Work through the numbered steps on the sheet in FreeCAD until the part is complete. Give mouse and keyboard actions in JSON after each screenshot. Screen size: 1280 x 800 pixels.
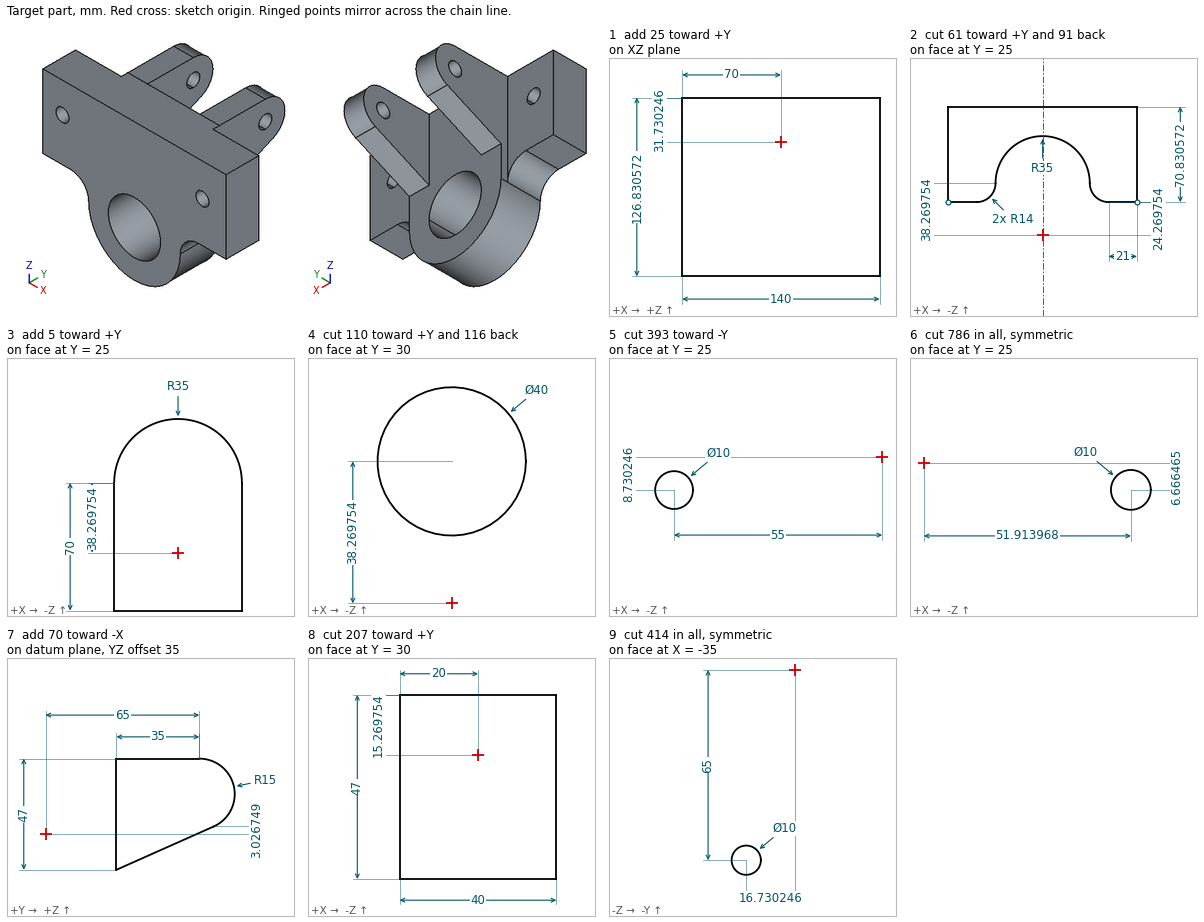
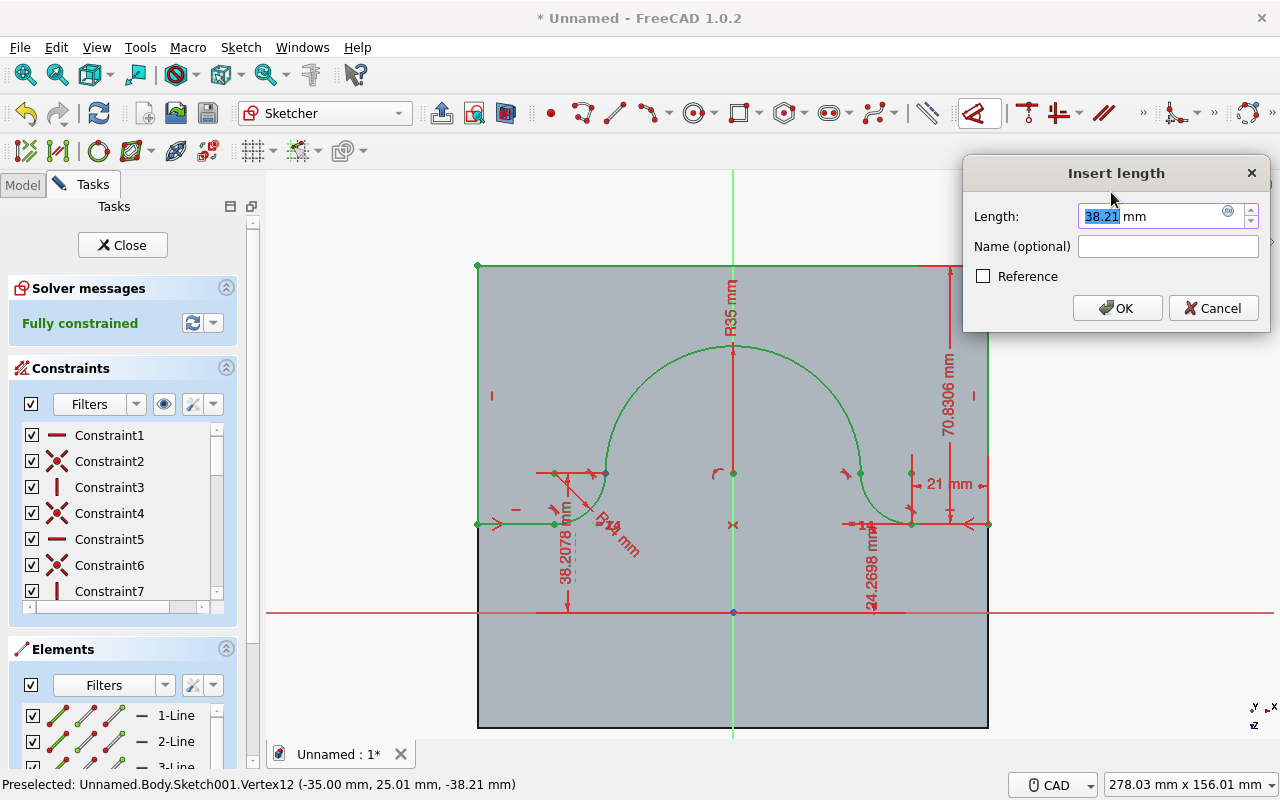
{"action": "type", "text": "38.269754"}
{"action": "key", "text": "Return"}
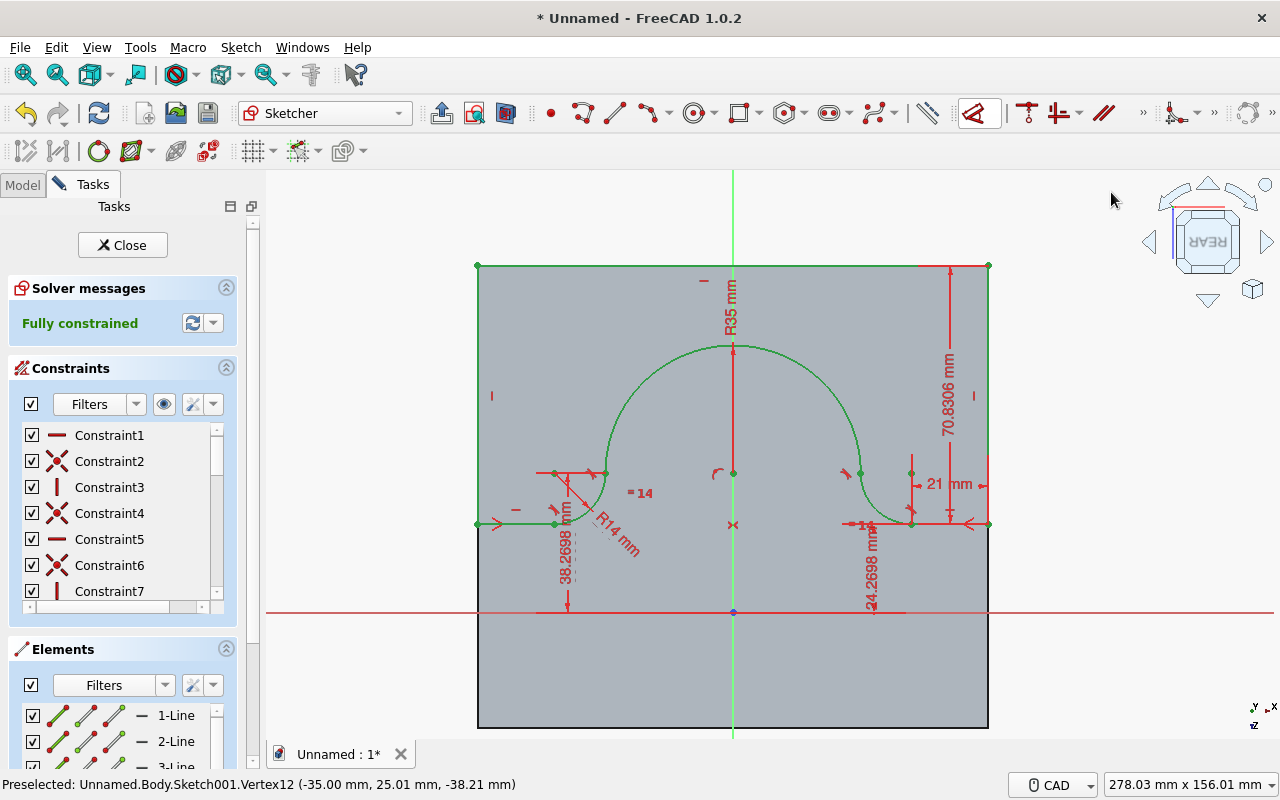
{"action": "left_click", "coordinate": [123, 245]}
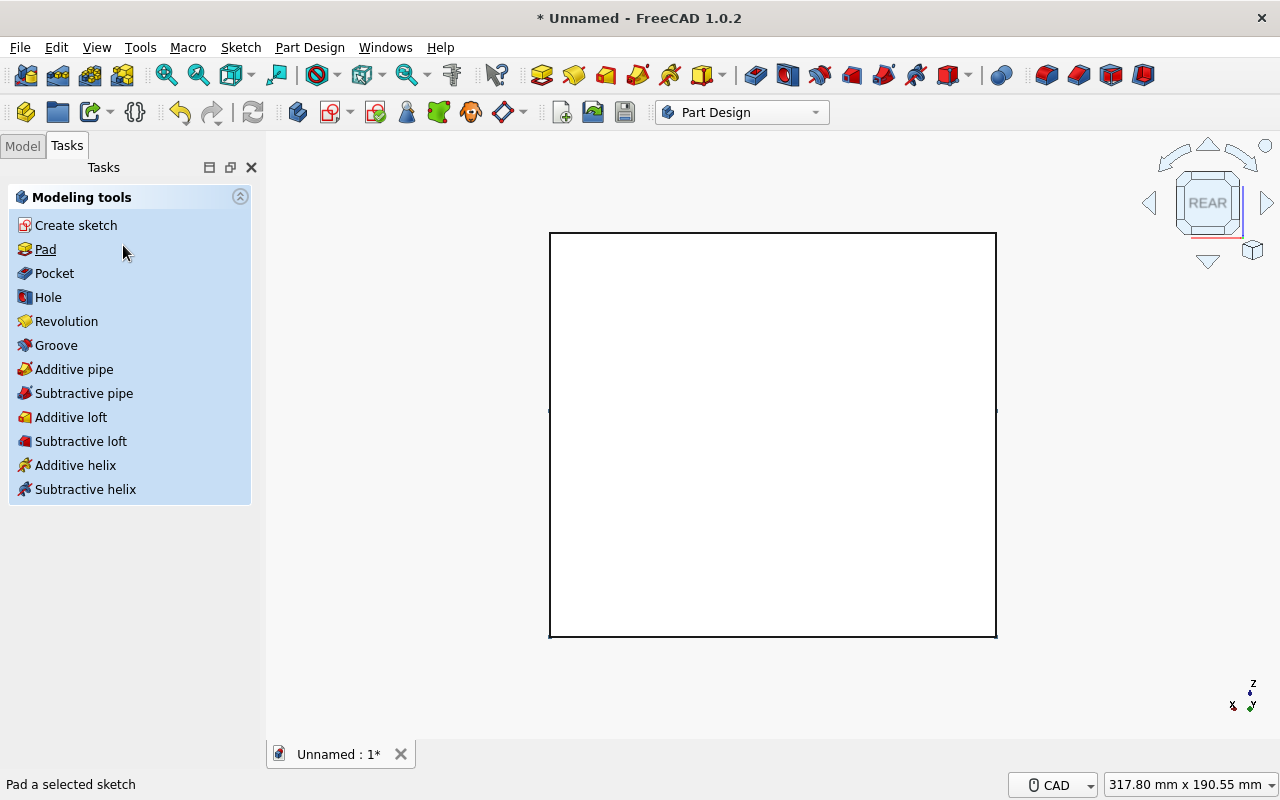
{"action": "left_click", "coordinate": [756, 76]}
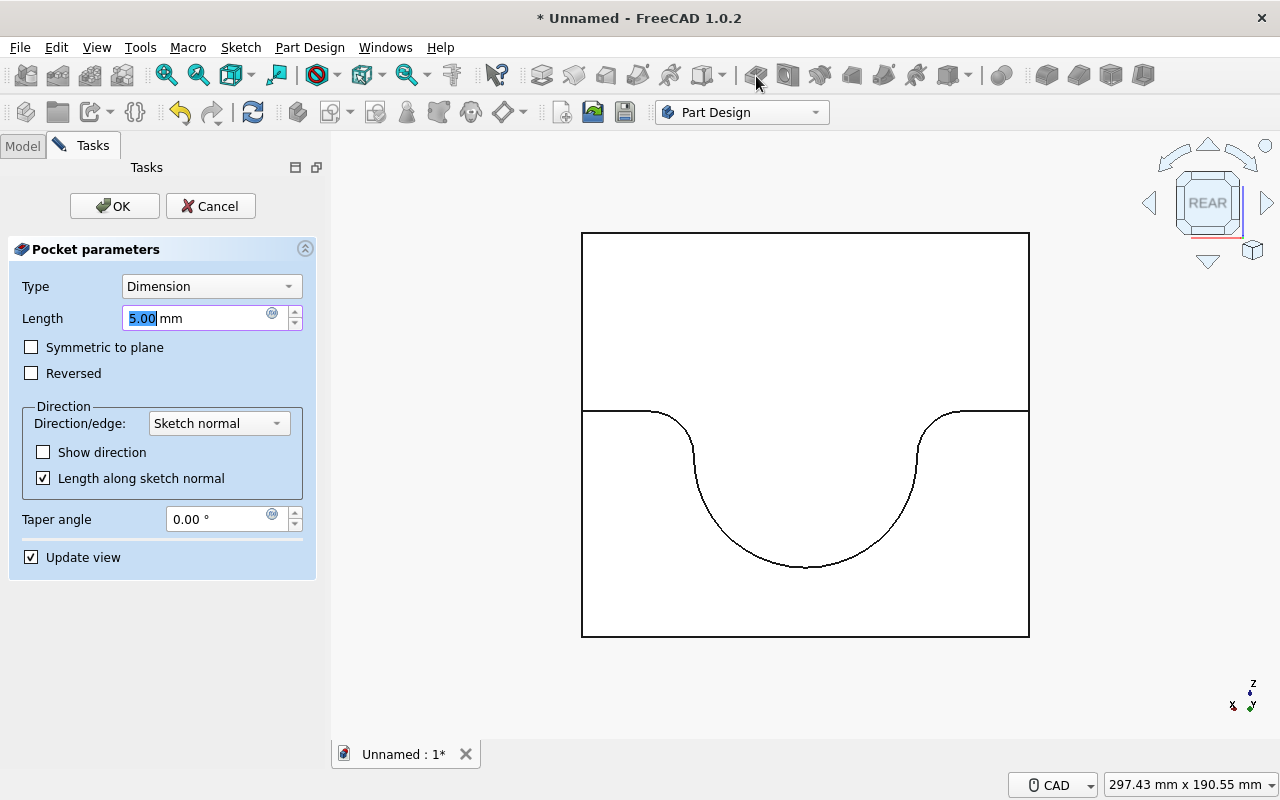
{"action": "left_click", "coordinate": [212, 286]}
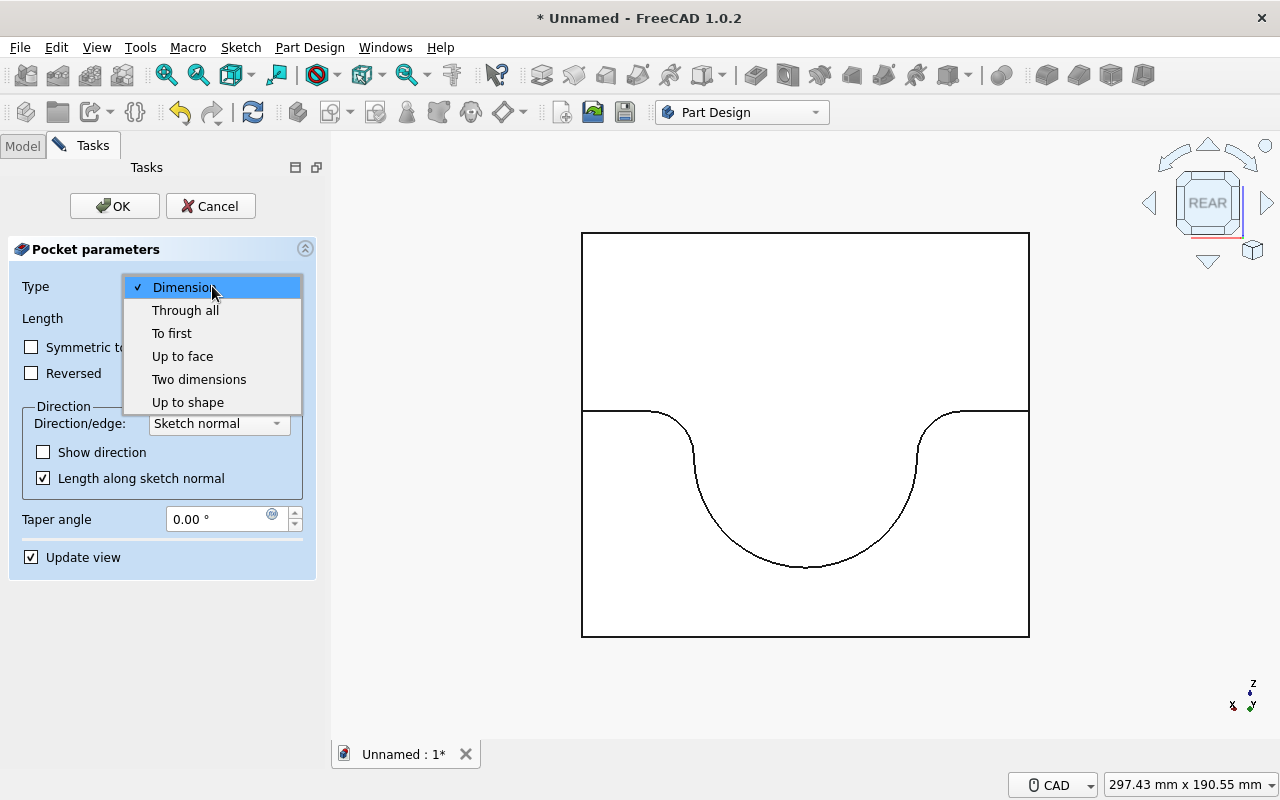
{"action": "left_click", "coordinate": [212, 380]}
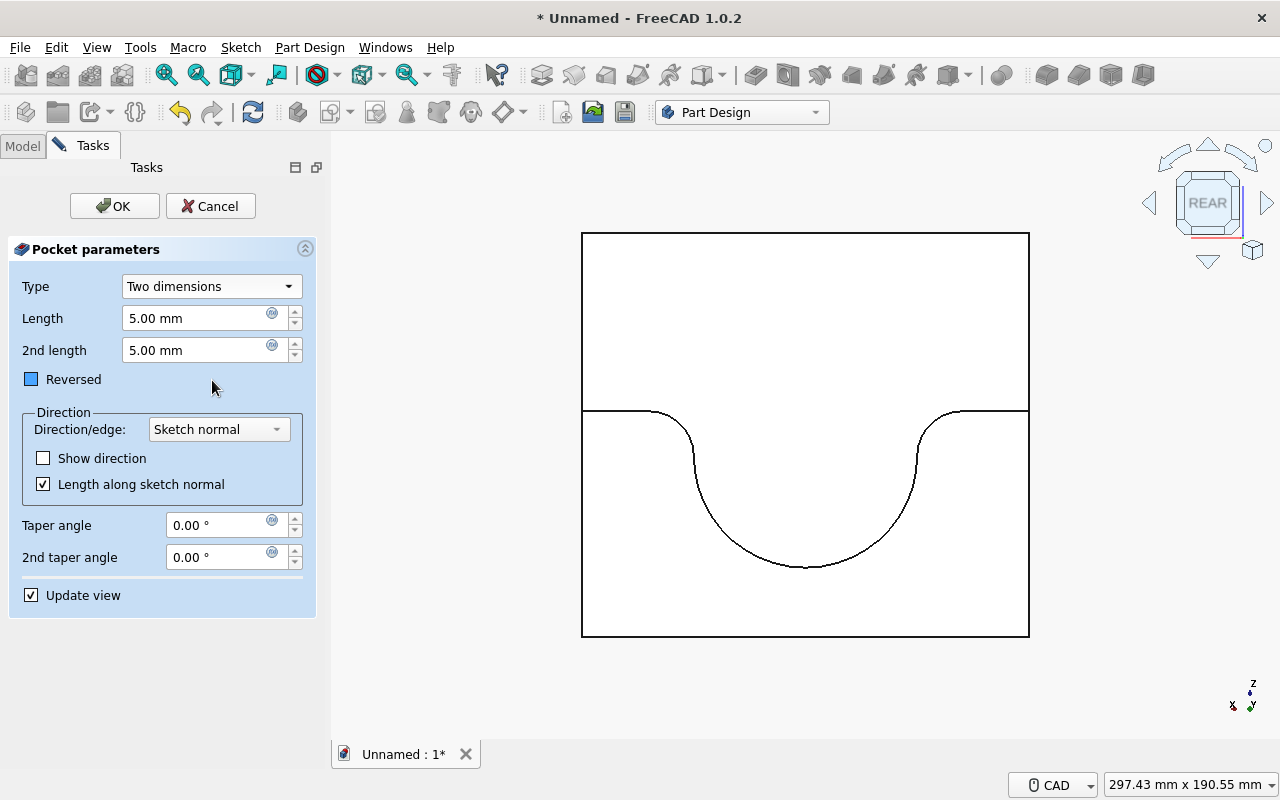
{"action": "triple_click", "coordinate": [204, 318]}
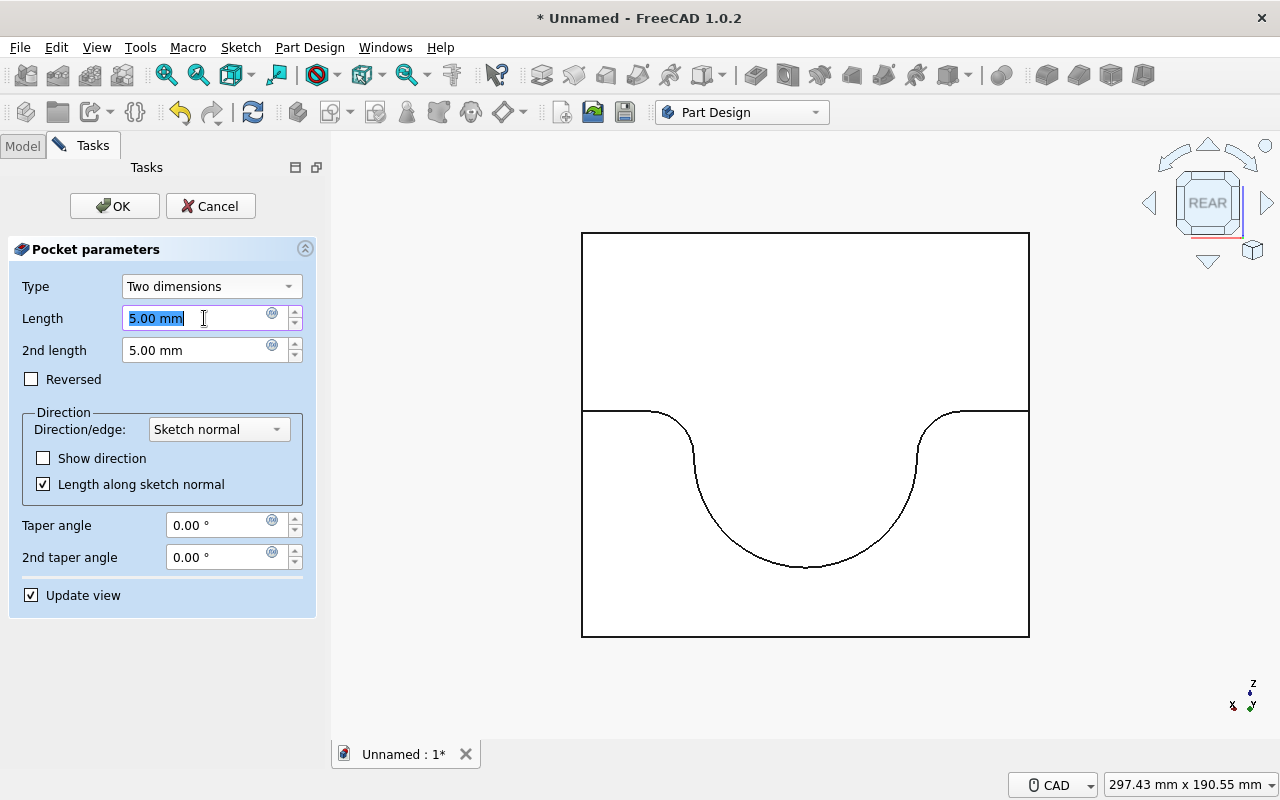
{"action": "type", "text": "61"}
{"action": "key", "text": "Tab"}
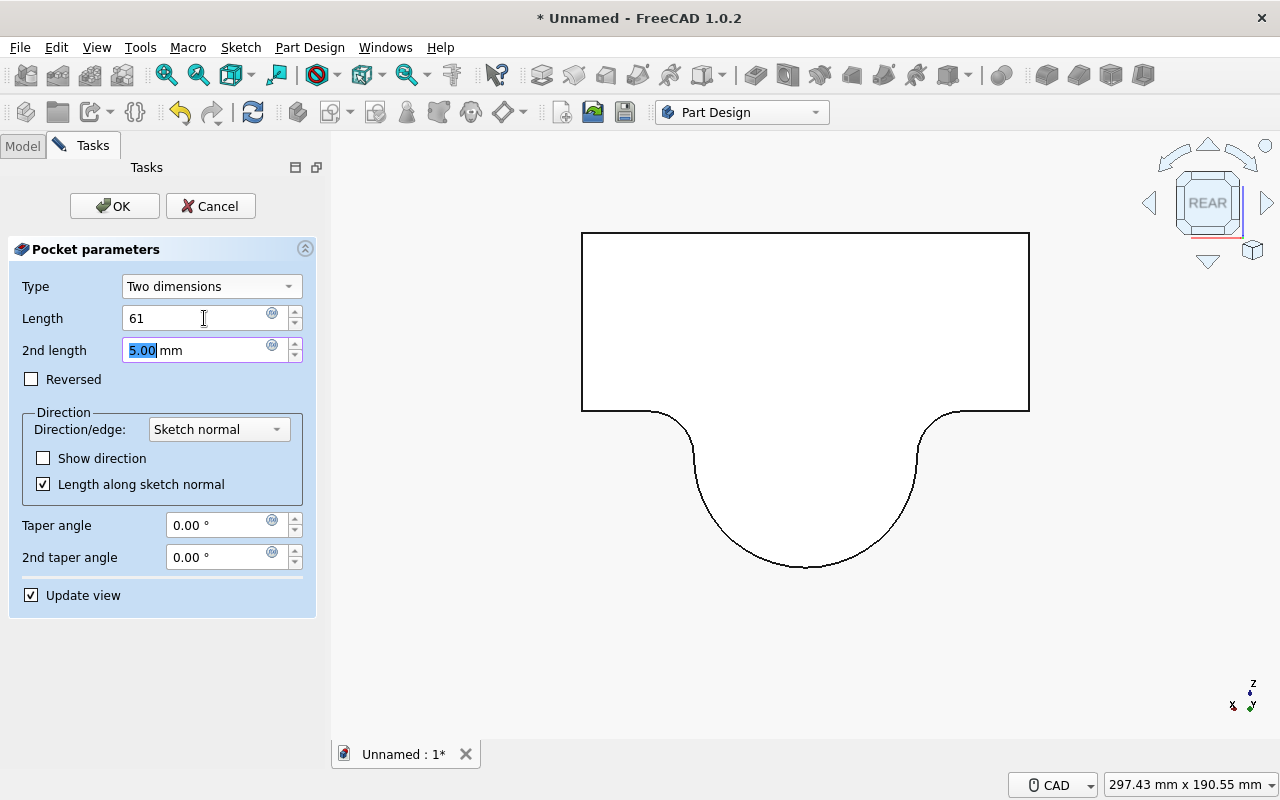
{"action": "type", "text": "91"}
{"action": "key", "text": "Tab"}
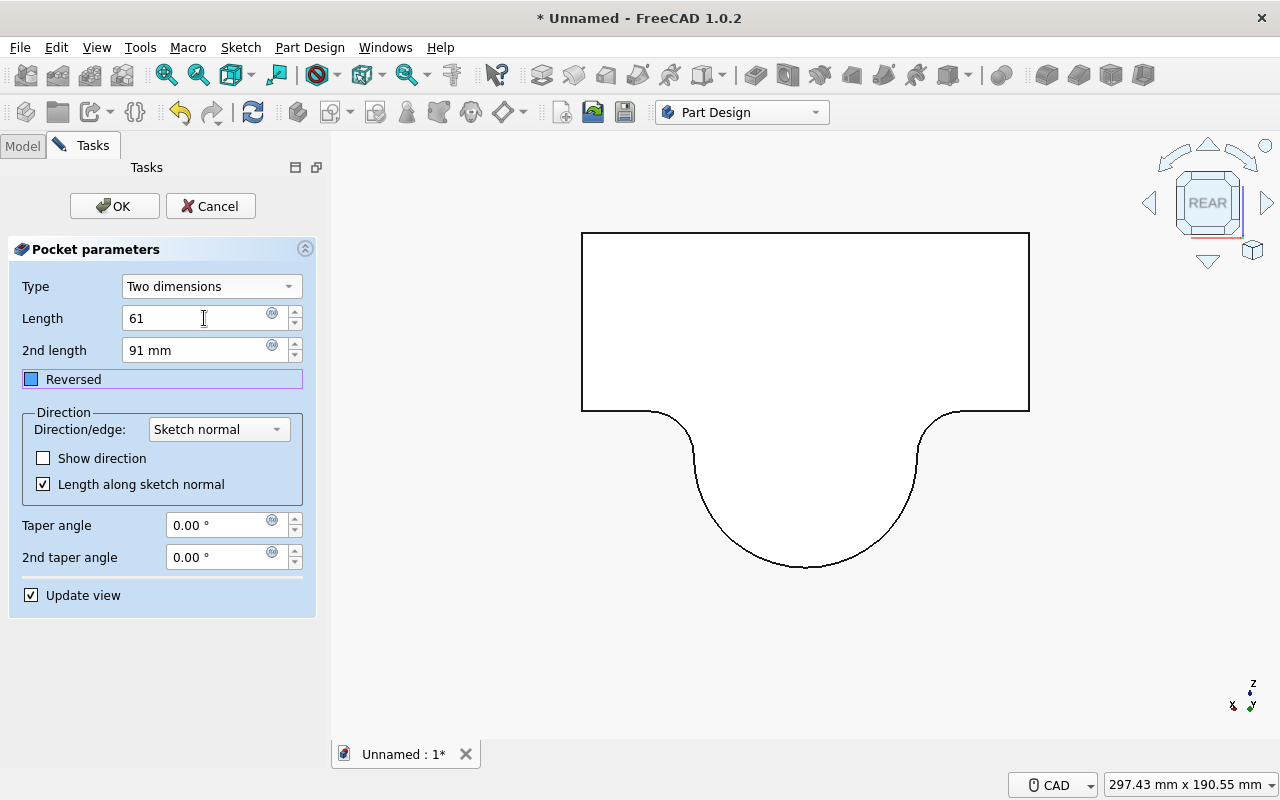
{"action": "left_click", "coordinate": [30, 379]}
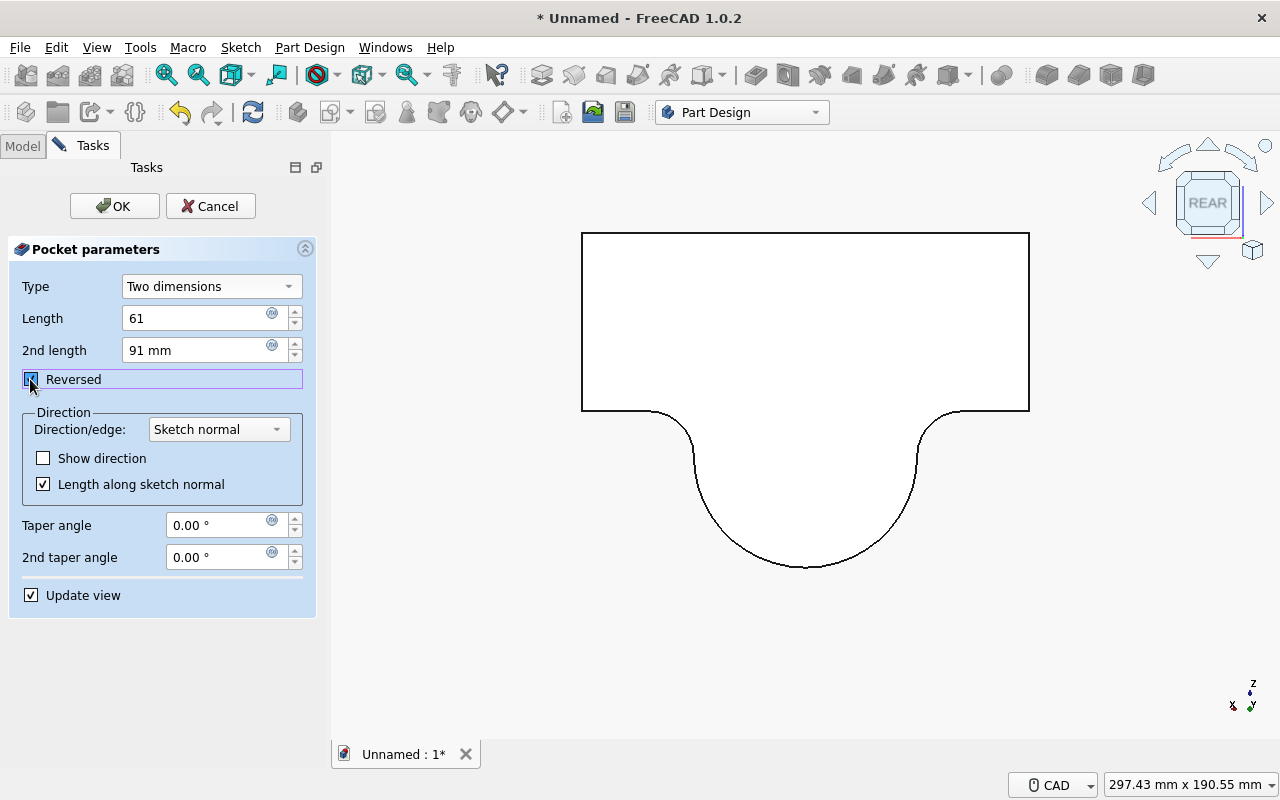
{"action": "left_click", "coordinate": [115, 206]}